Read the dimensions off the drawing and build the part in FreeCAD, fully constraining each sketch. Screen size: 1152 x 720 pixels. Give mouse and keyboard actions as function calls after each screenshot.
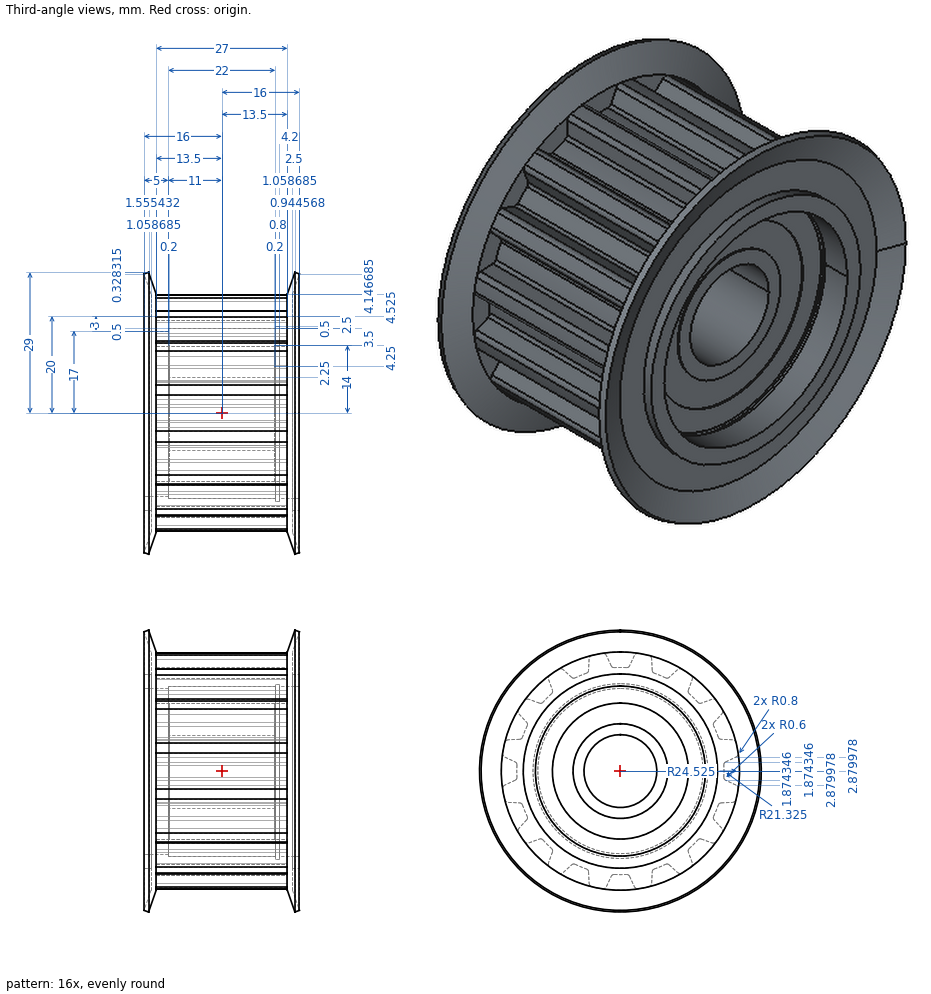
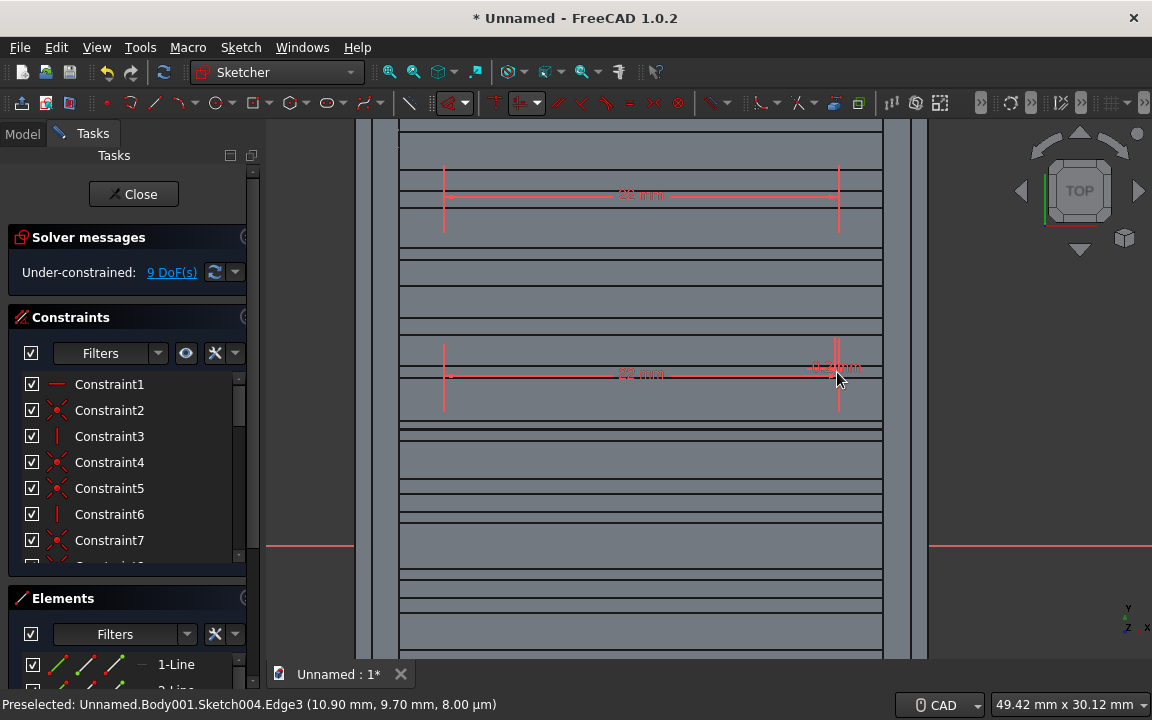
scroll(836, 296, up, 13)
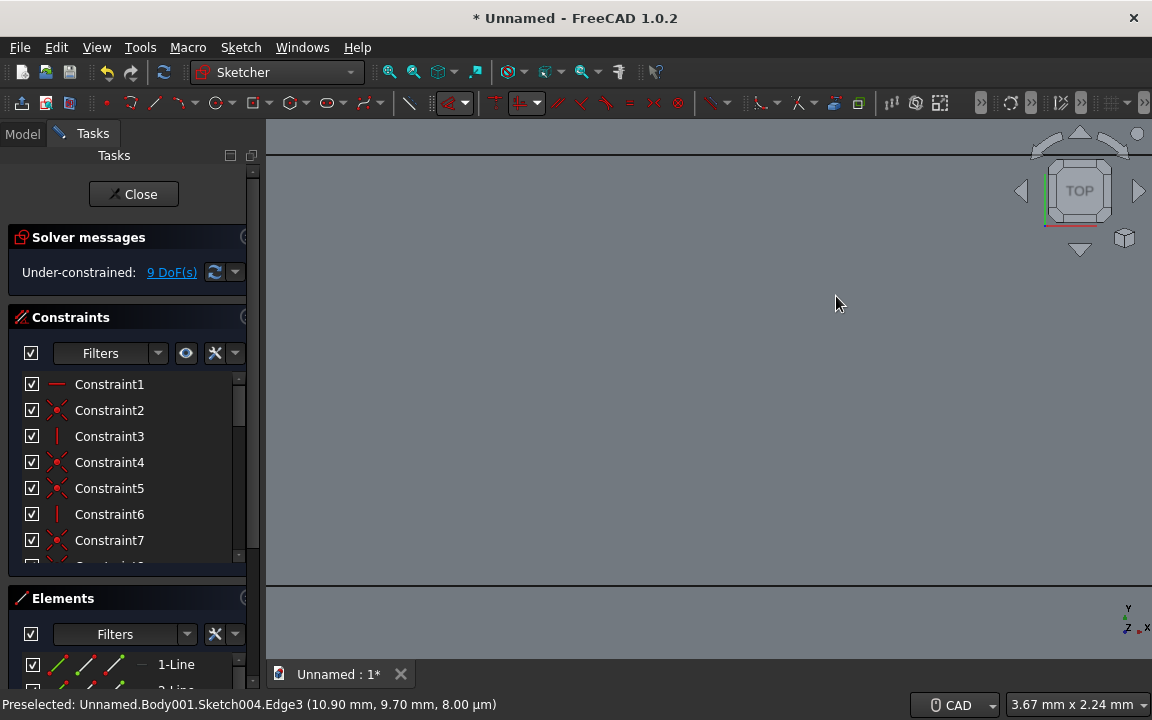
click(830, 292)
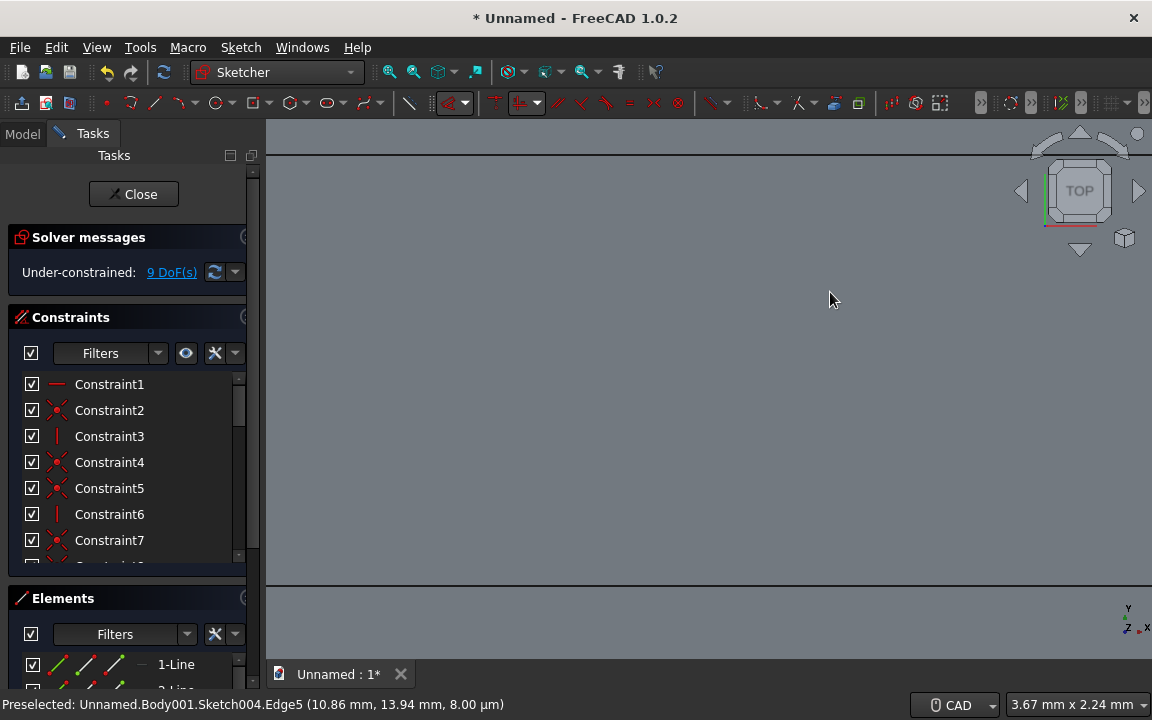
click(468, 104)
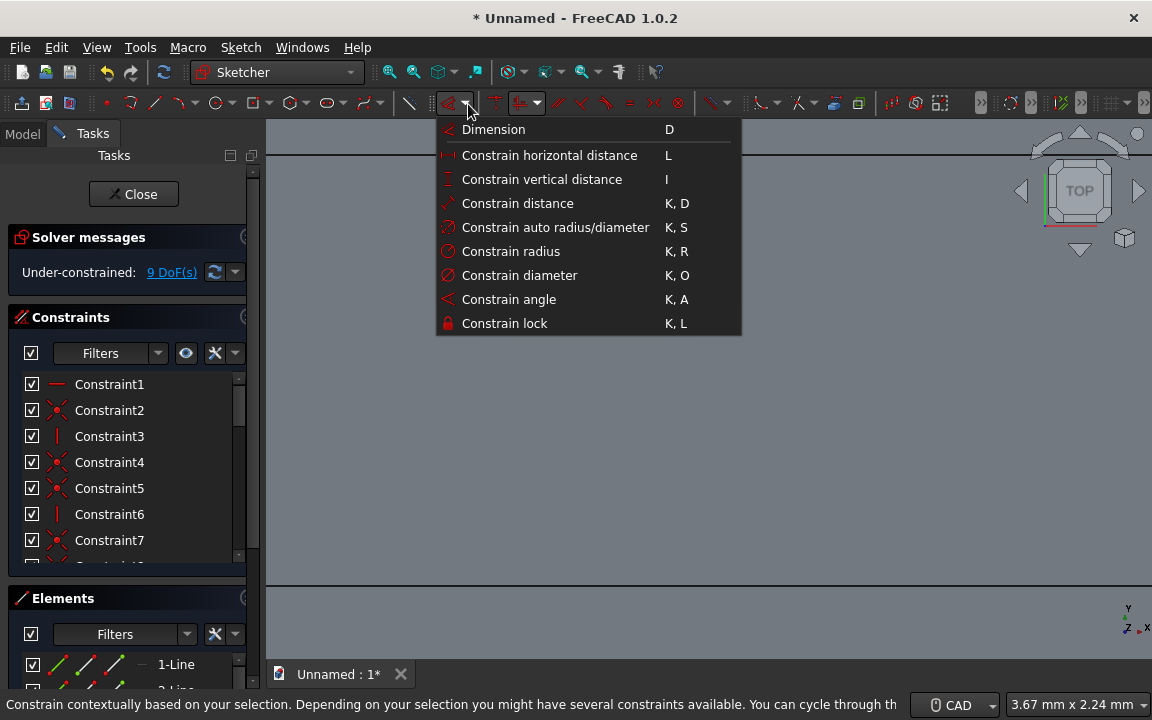
click(589, 155)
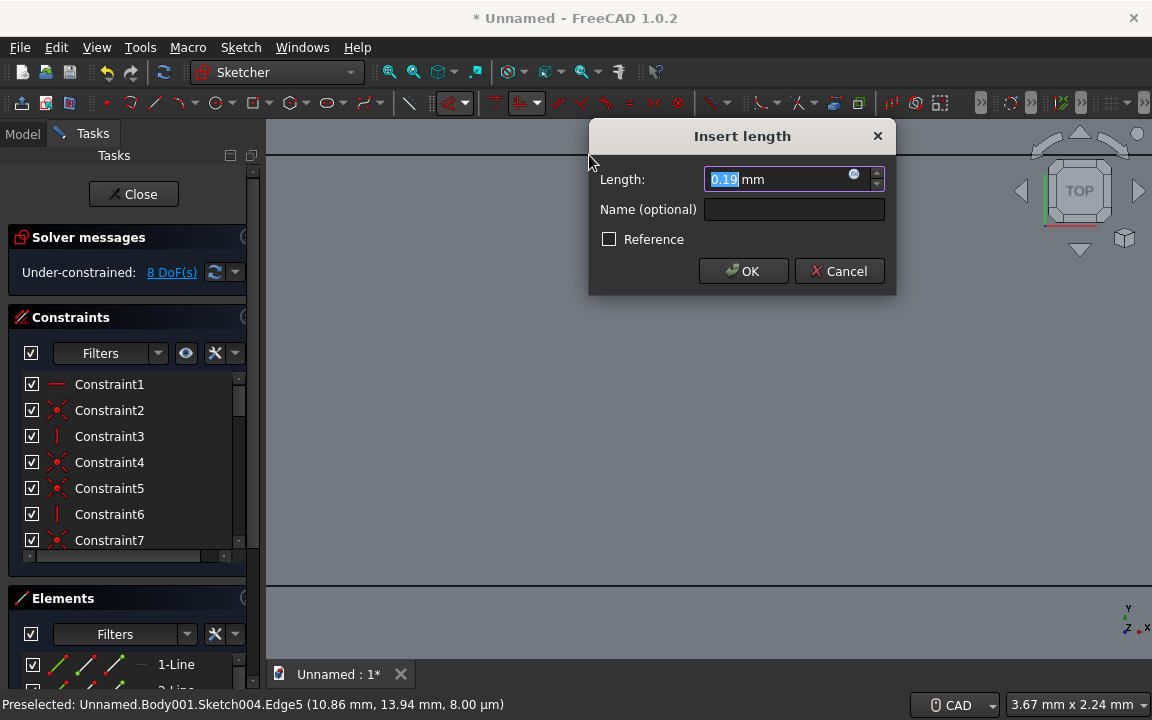
text(0.2)
key(Return)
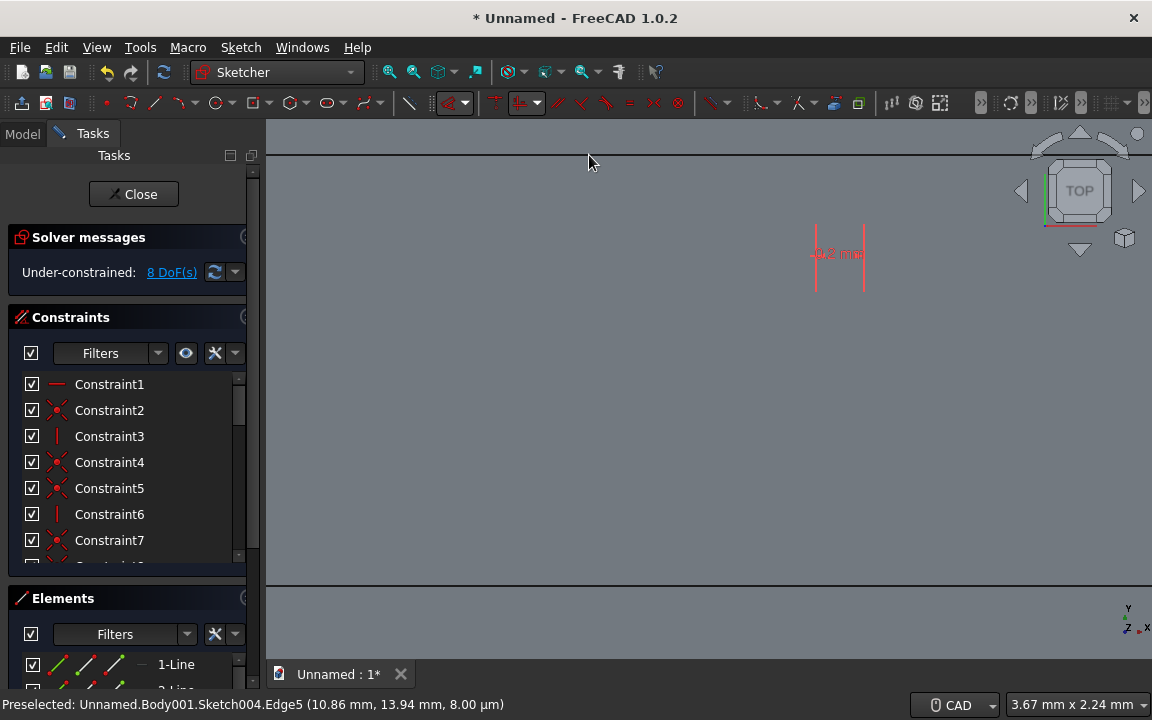
scroll(836, 296, down, 13)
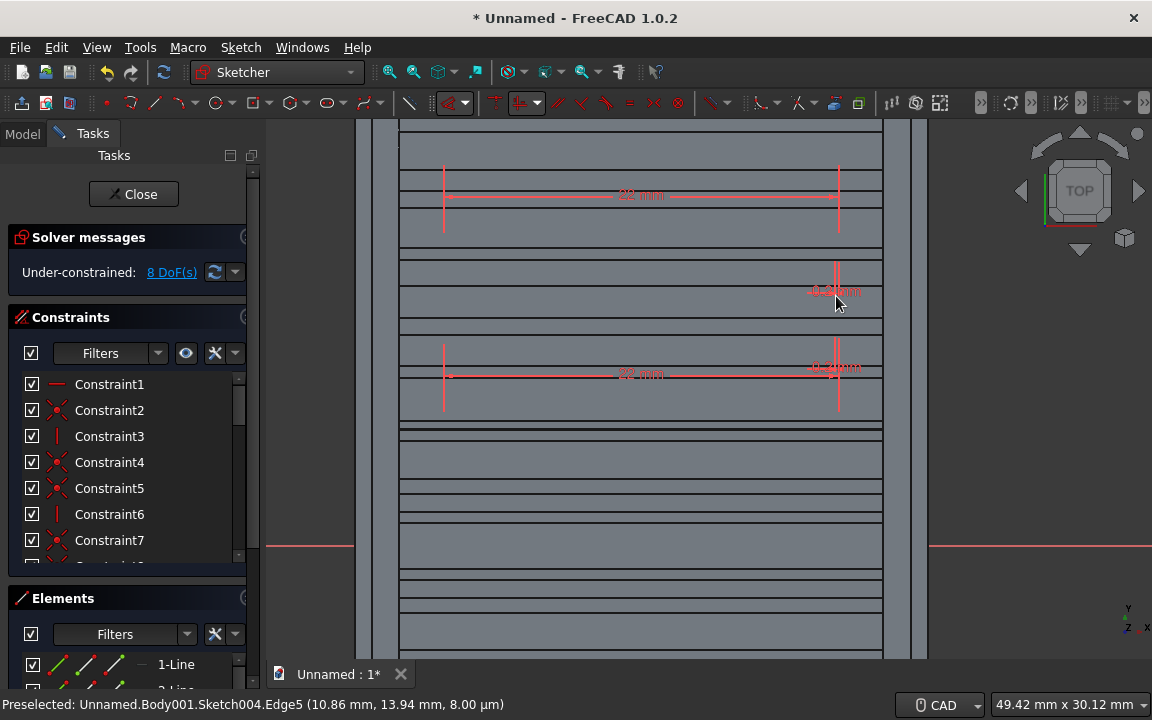
click(839, 252)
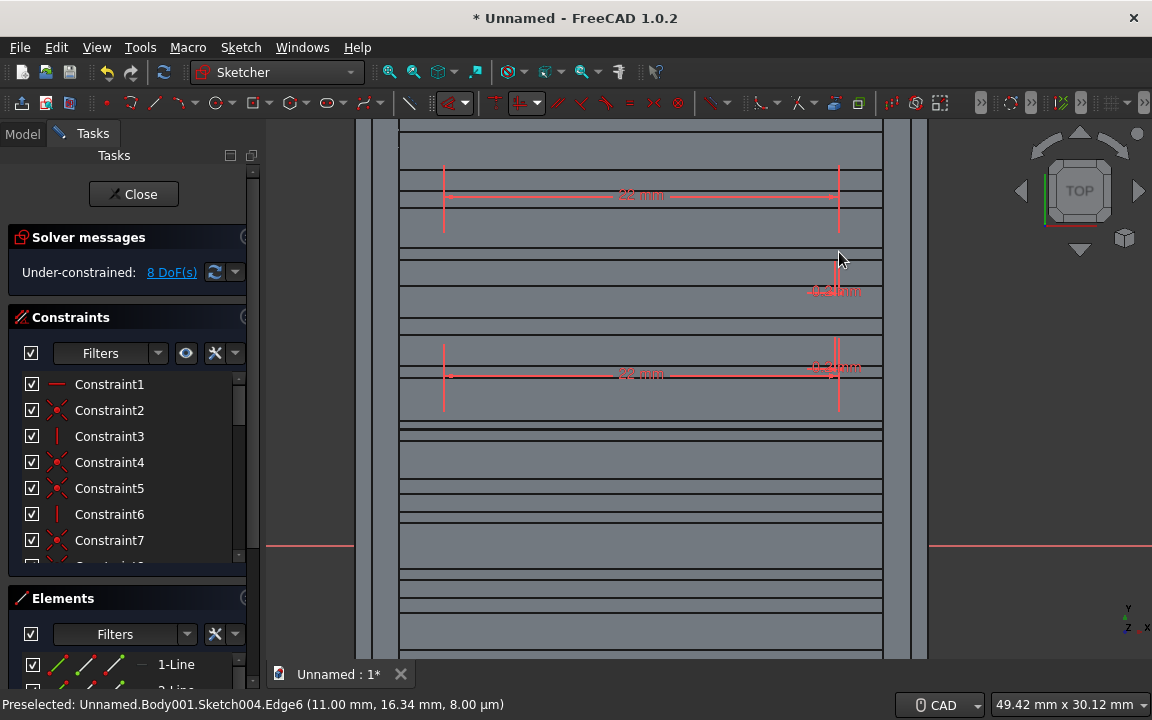
click(468, 104)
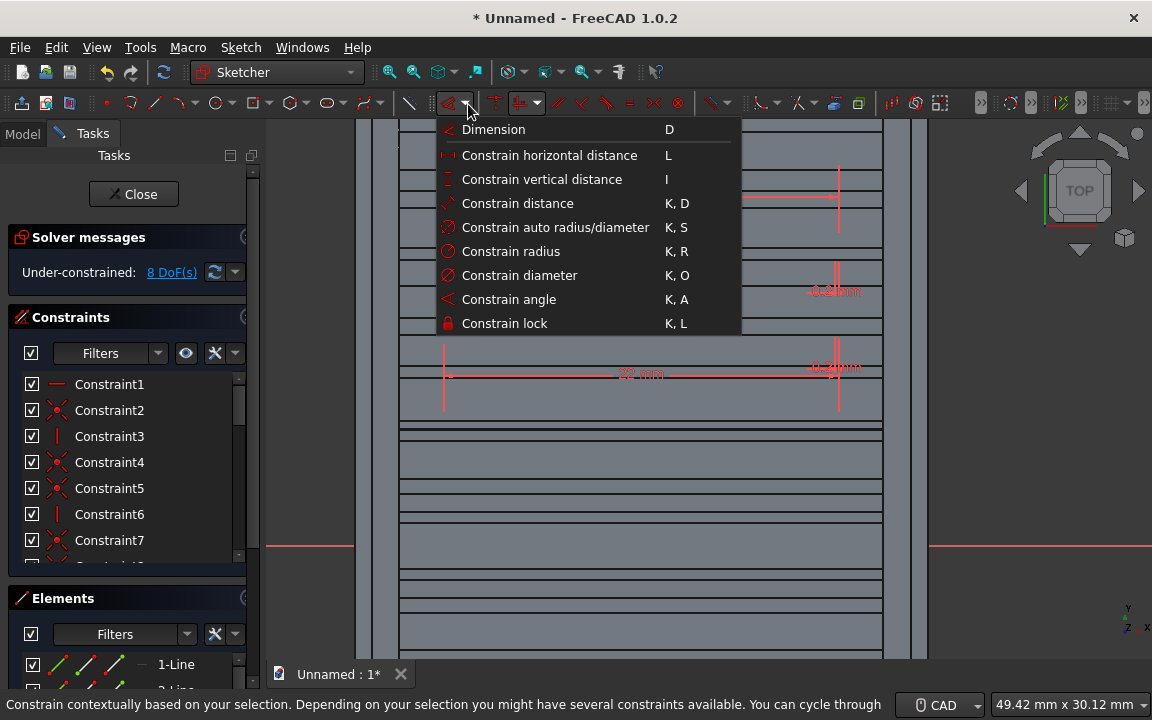
click(589, 179)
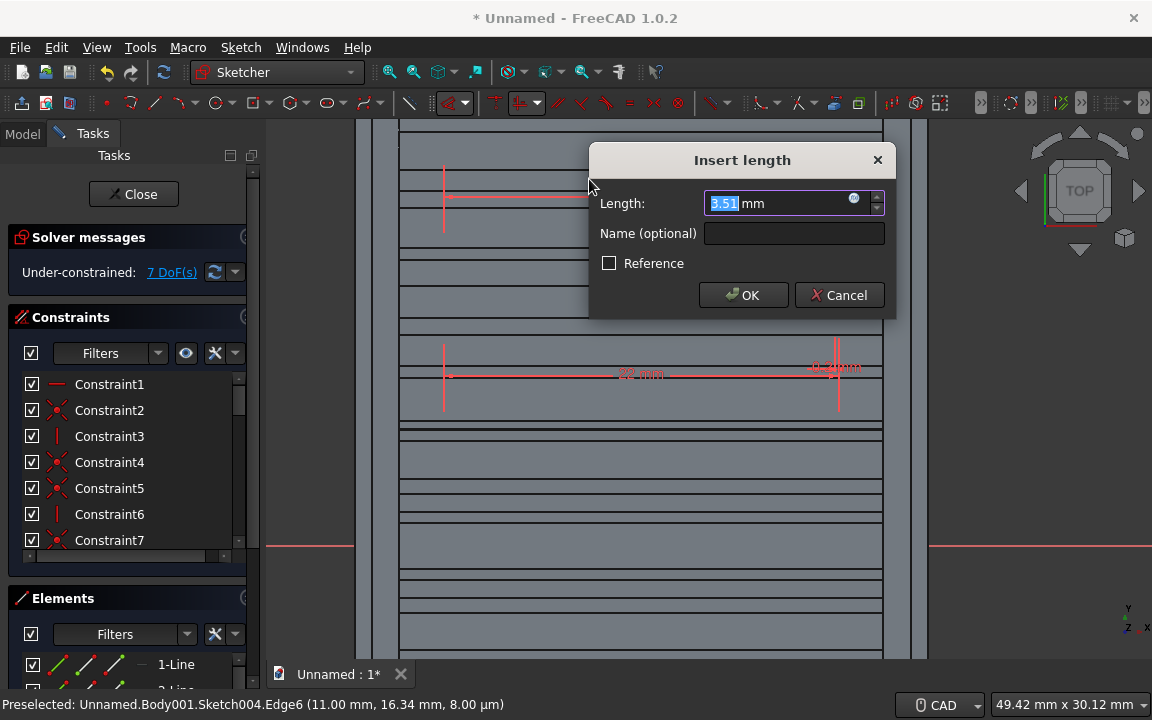
text(3.5)
key(Return)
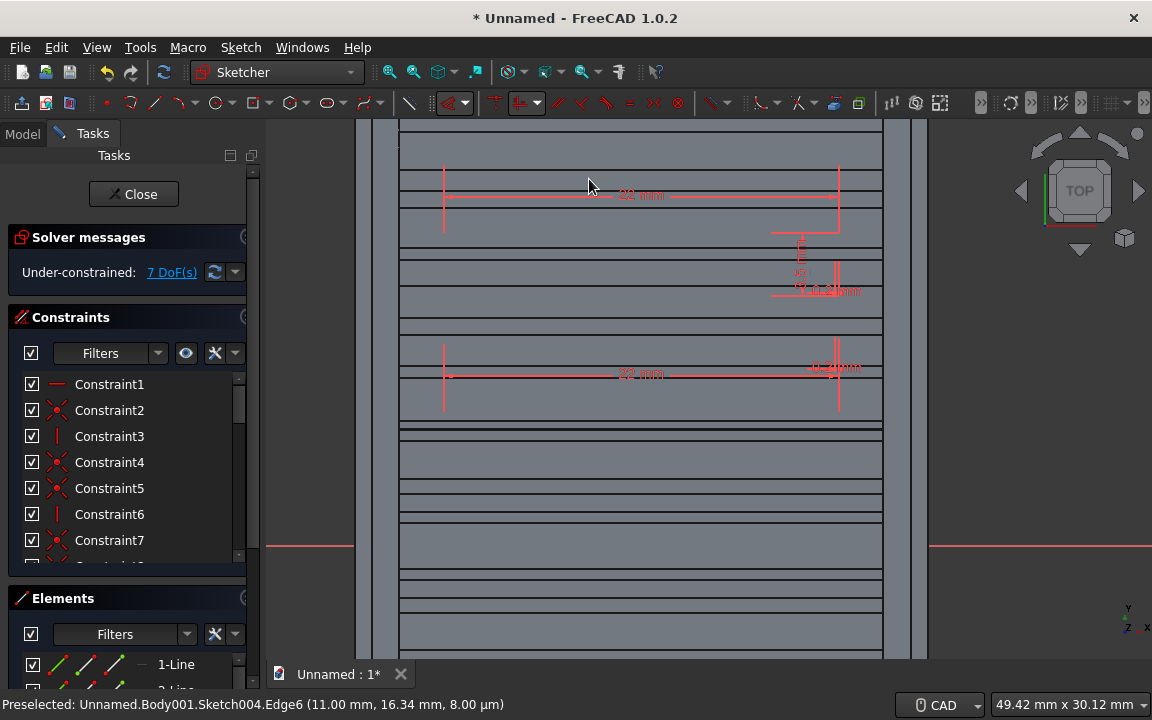
click(444, 252)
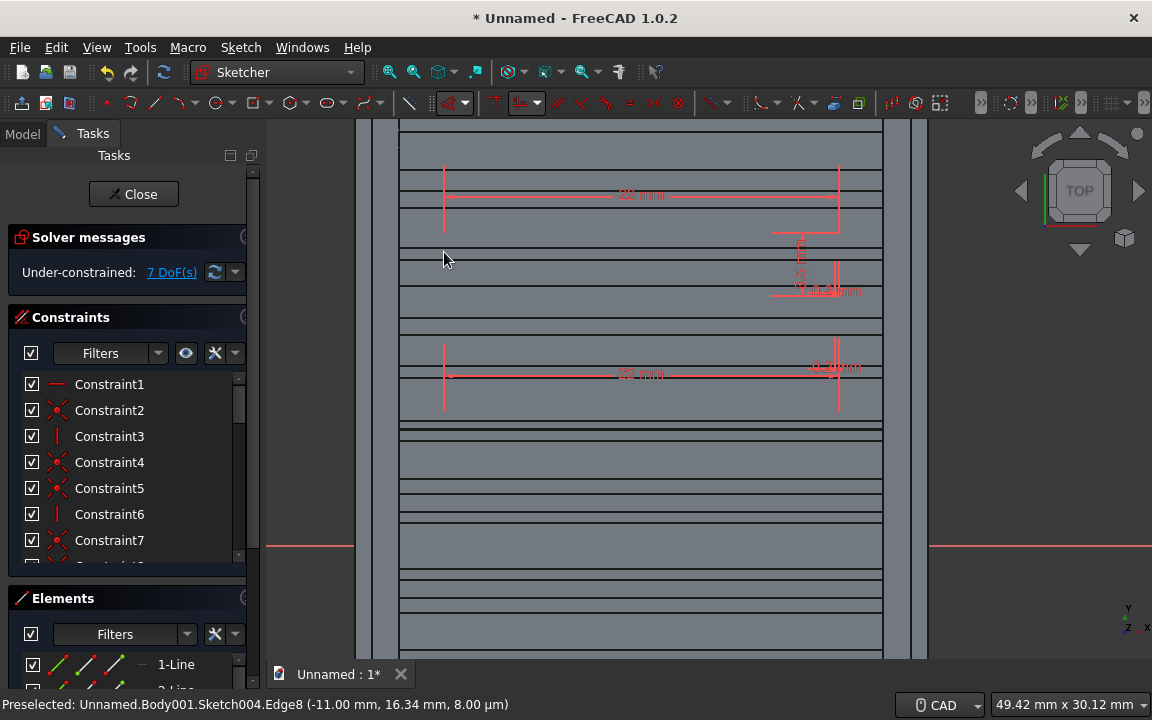
key(i)